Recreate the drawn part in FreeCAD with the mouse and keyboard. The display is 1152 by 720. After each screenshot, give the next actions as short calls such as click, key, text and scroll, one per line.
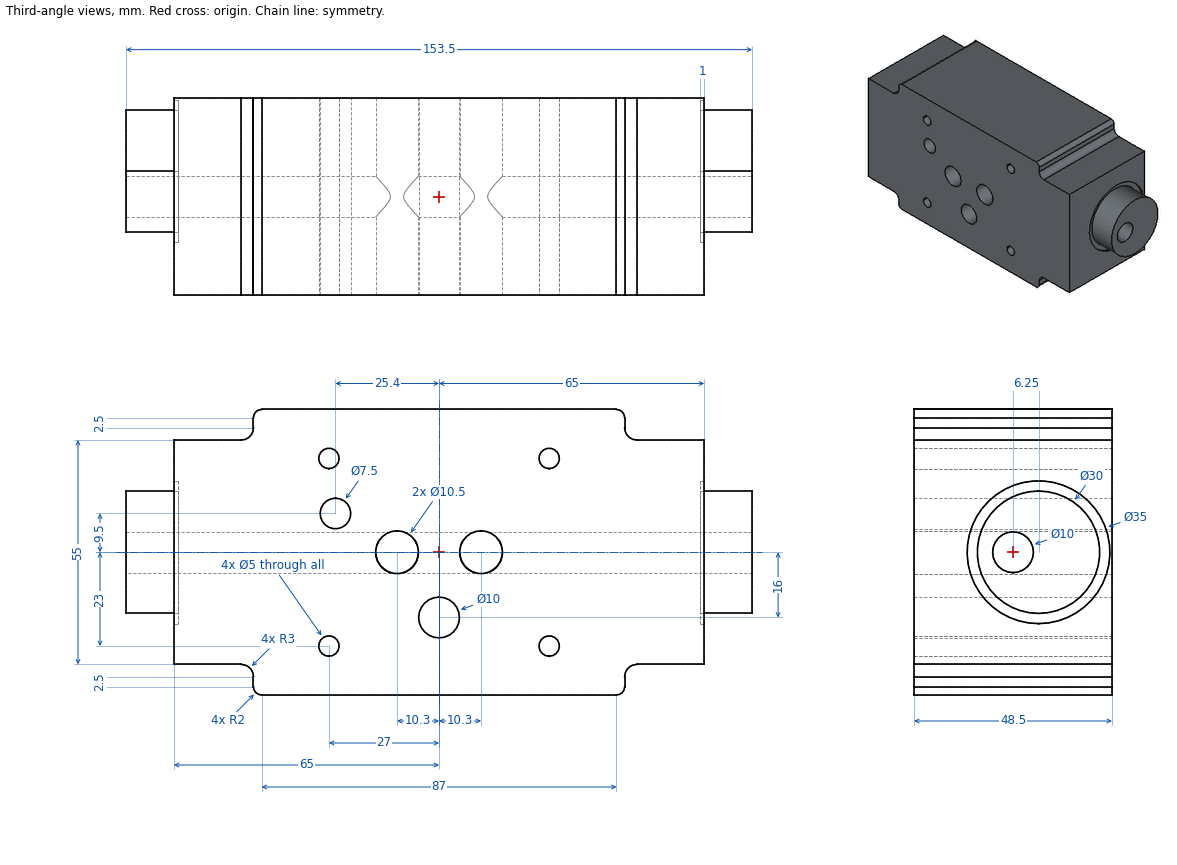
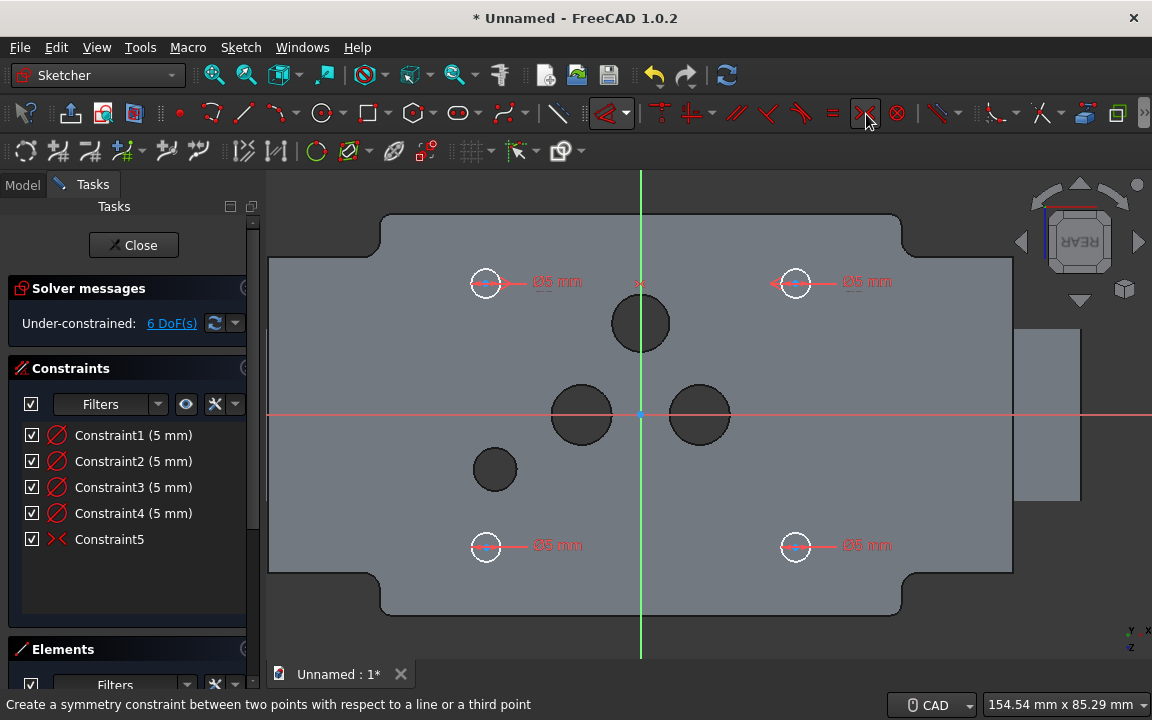
click(796, 284)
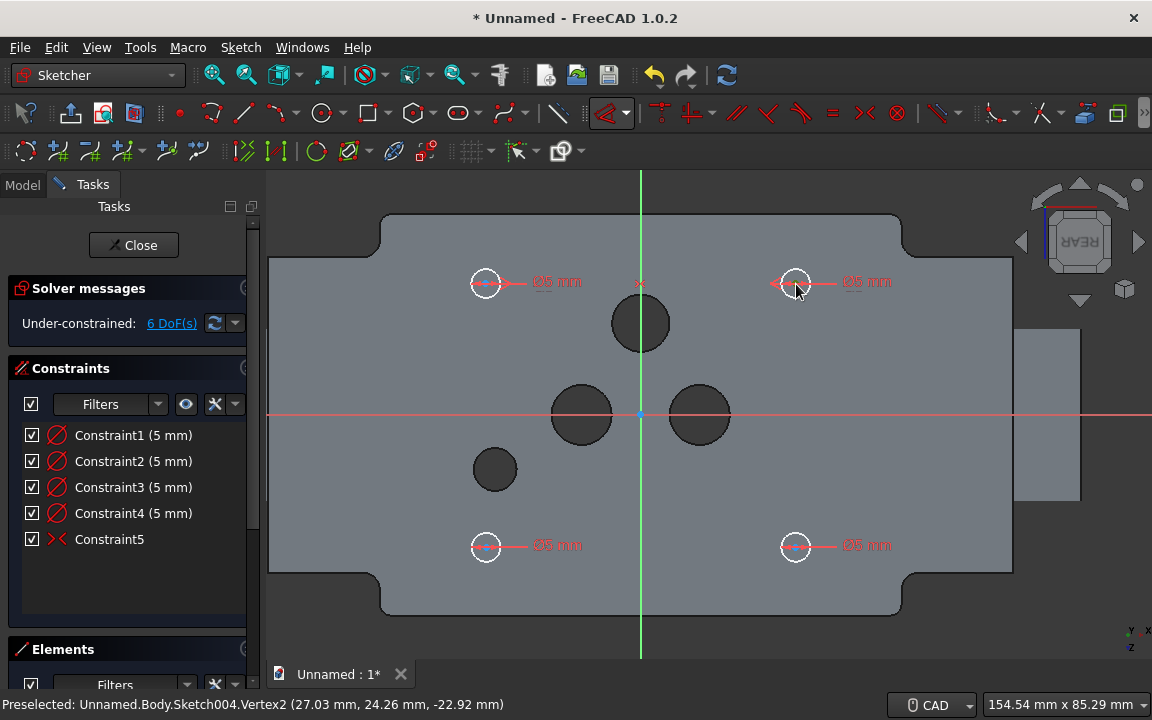
click(796, 547)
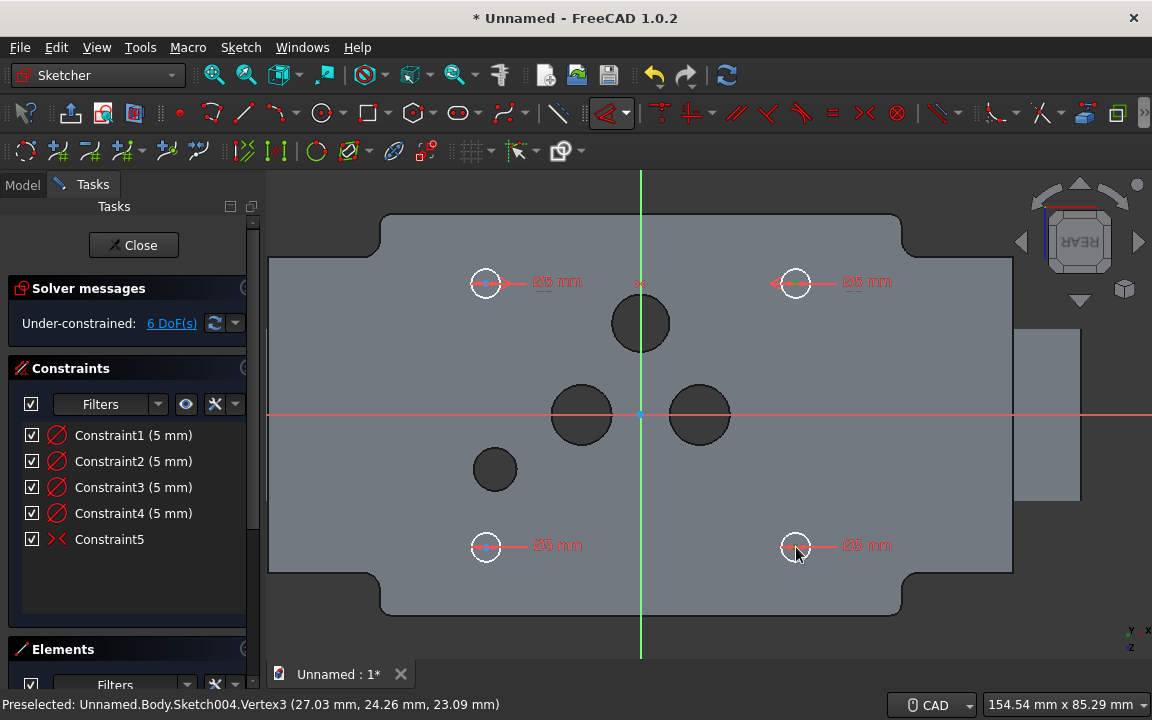
click(344, 415)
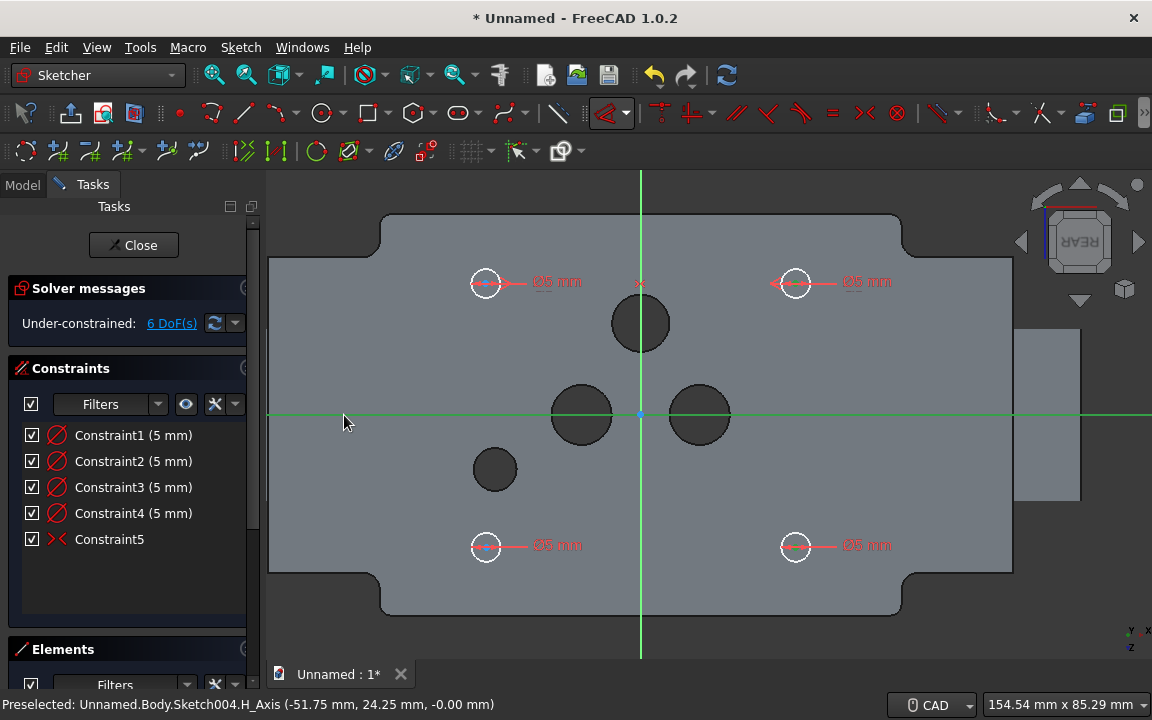
click(866, 114)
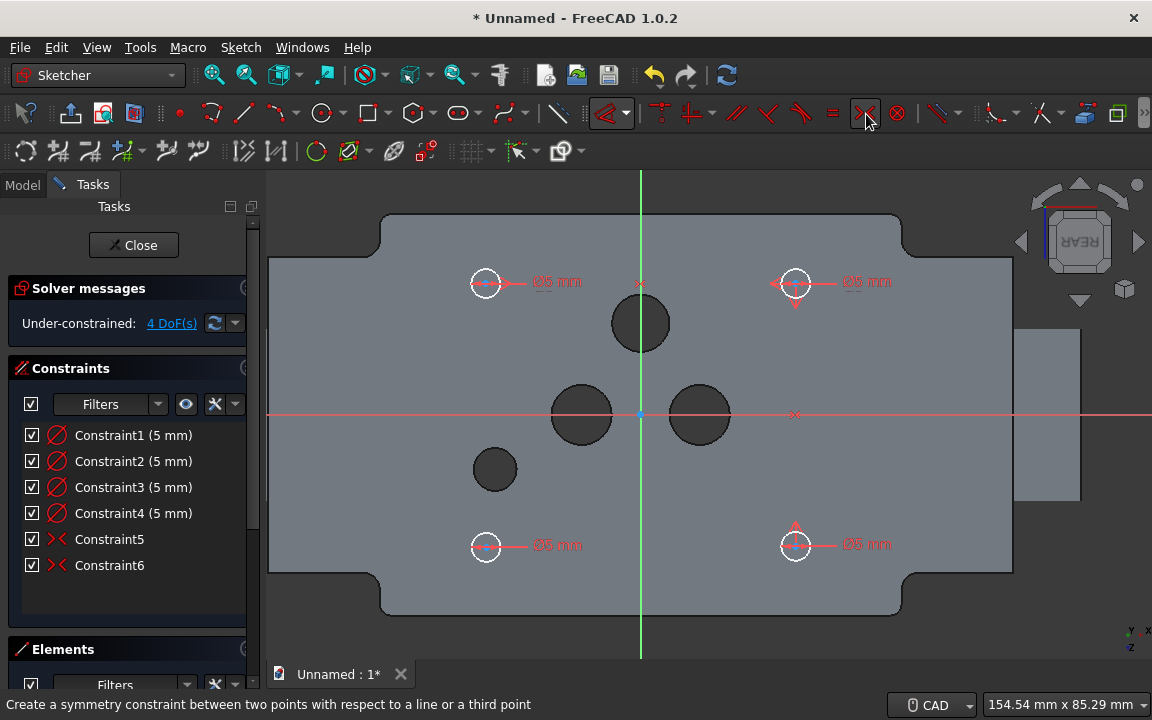
click(486, 284)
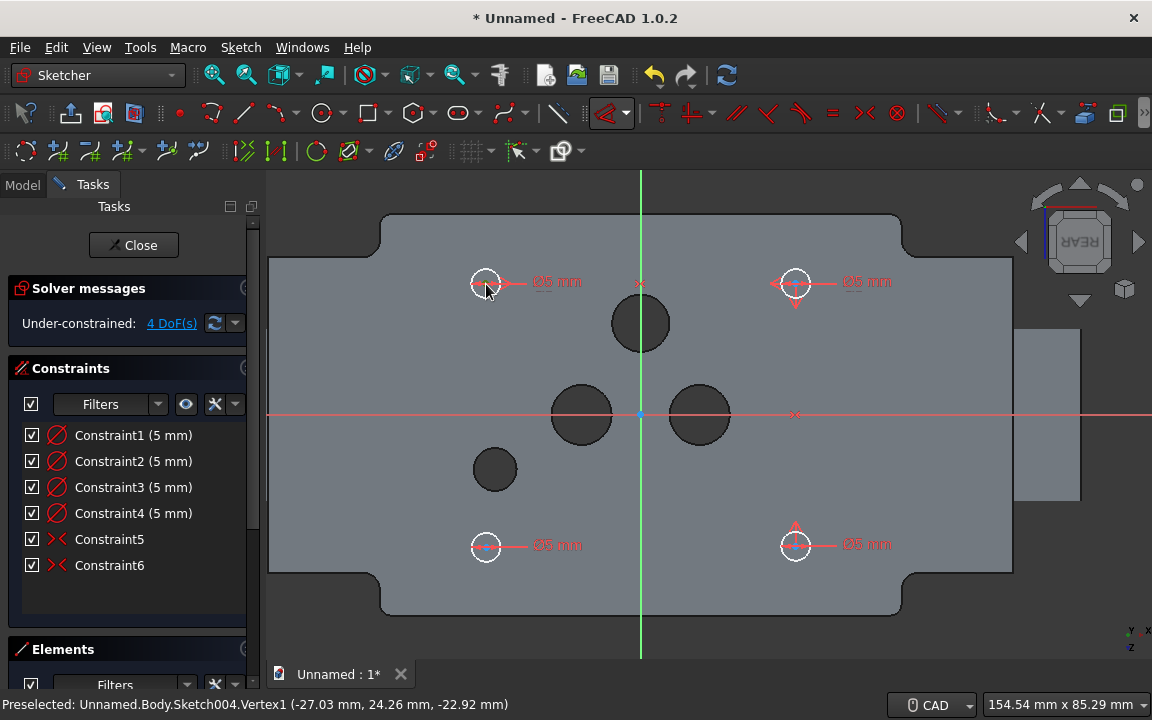
click(486, 547)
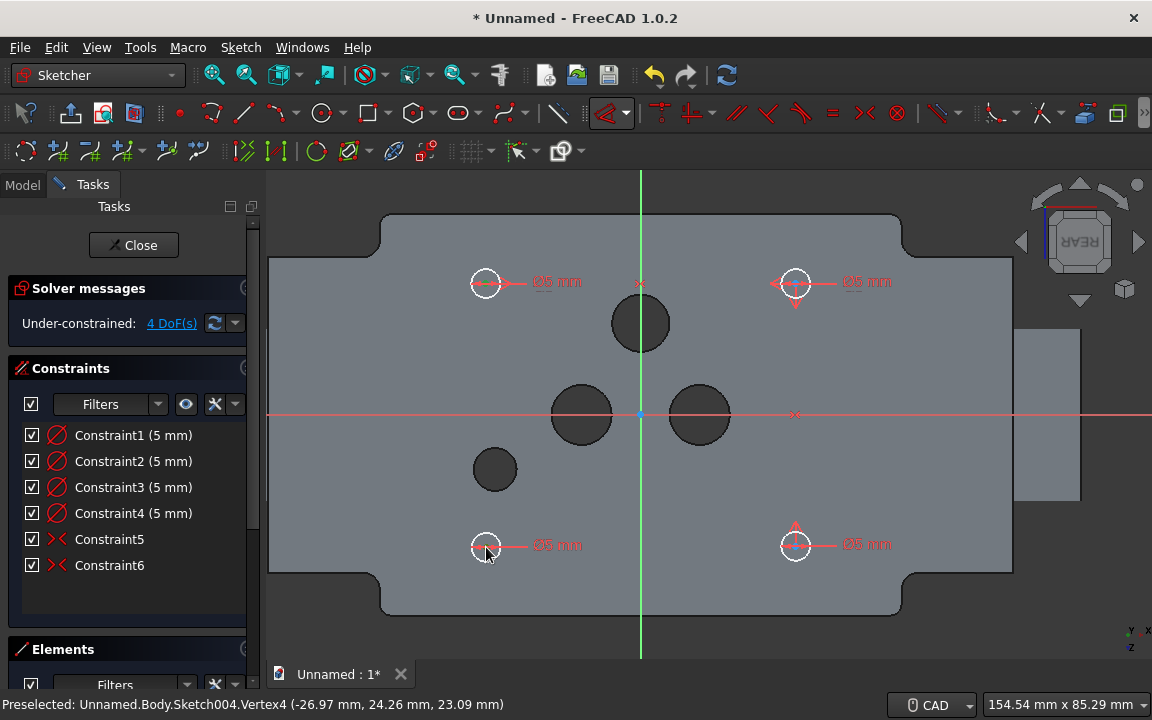
click(344, 415)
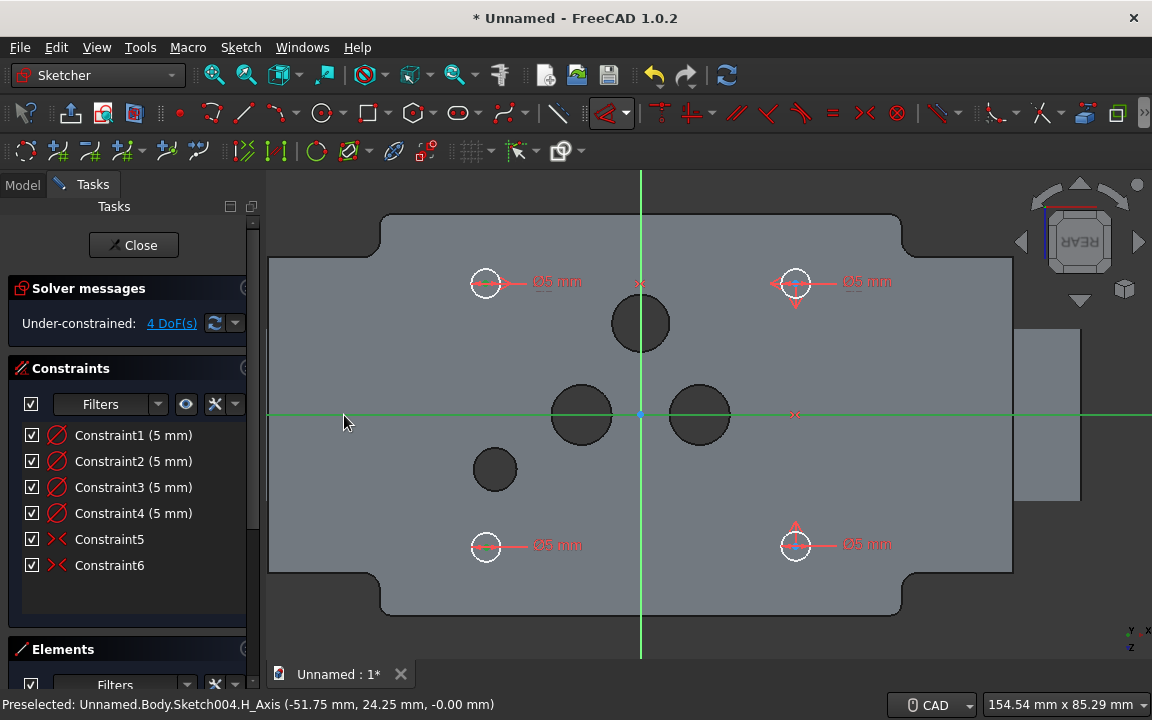
click(866, 114)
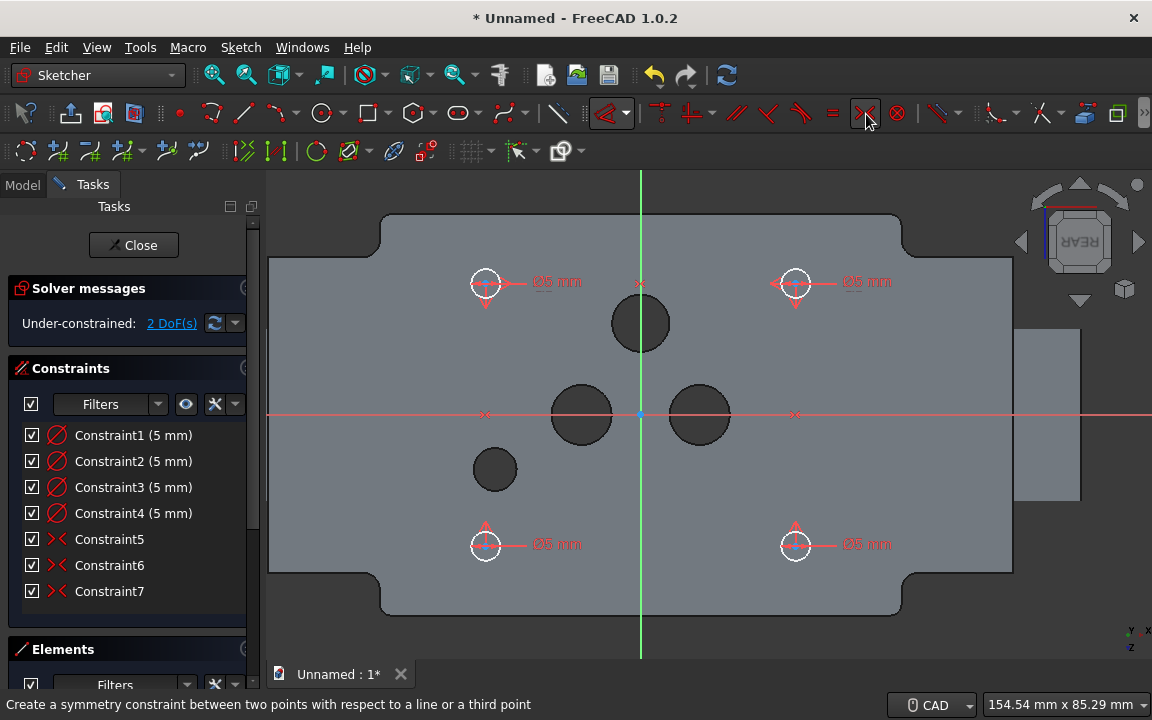
click(486, 284)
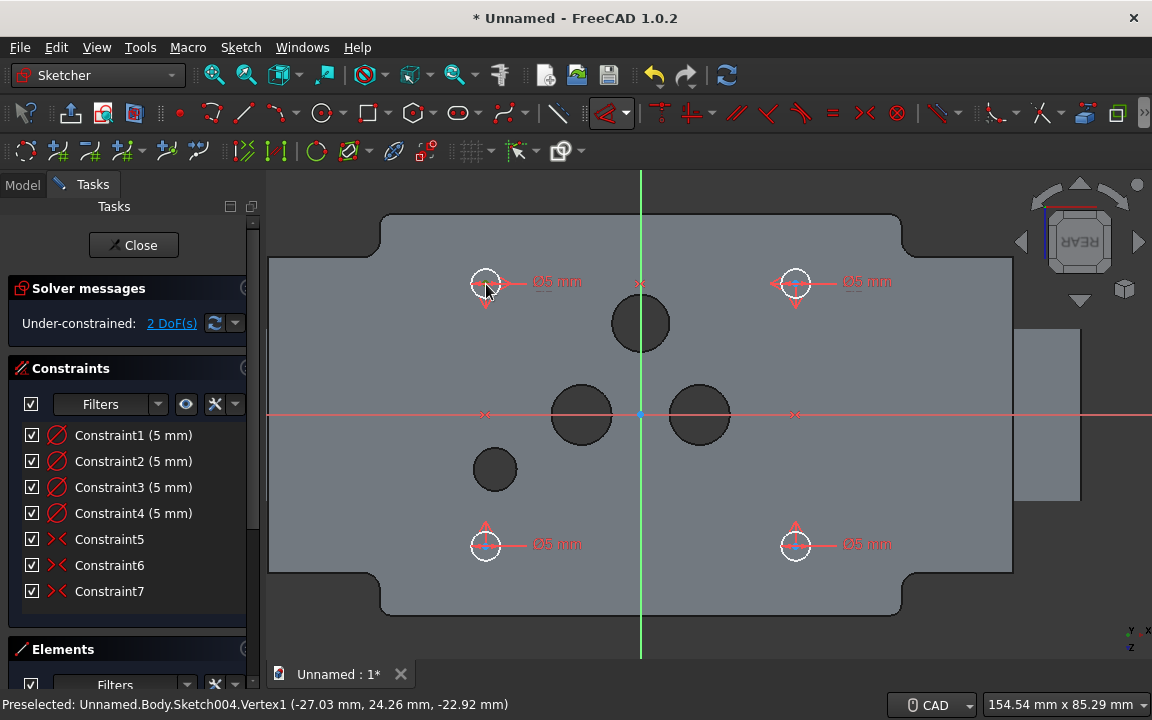
click(628, 114)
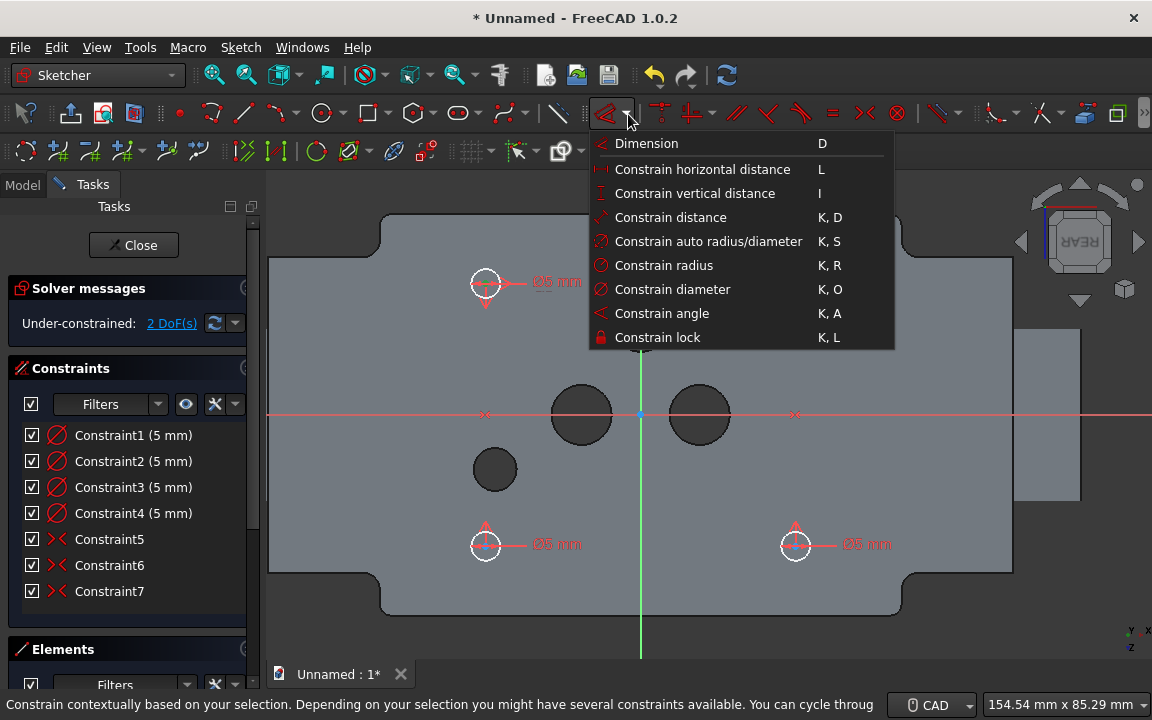
click(742, 169)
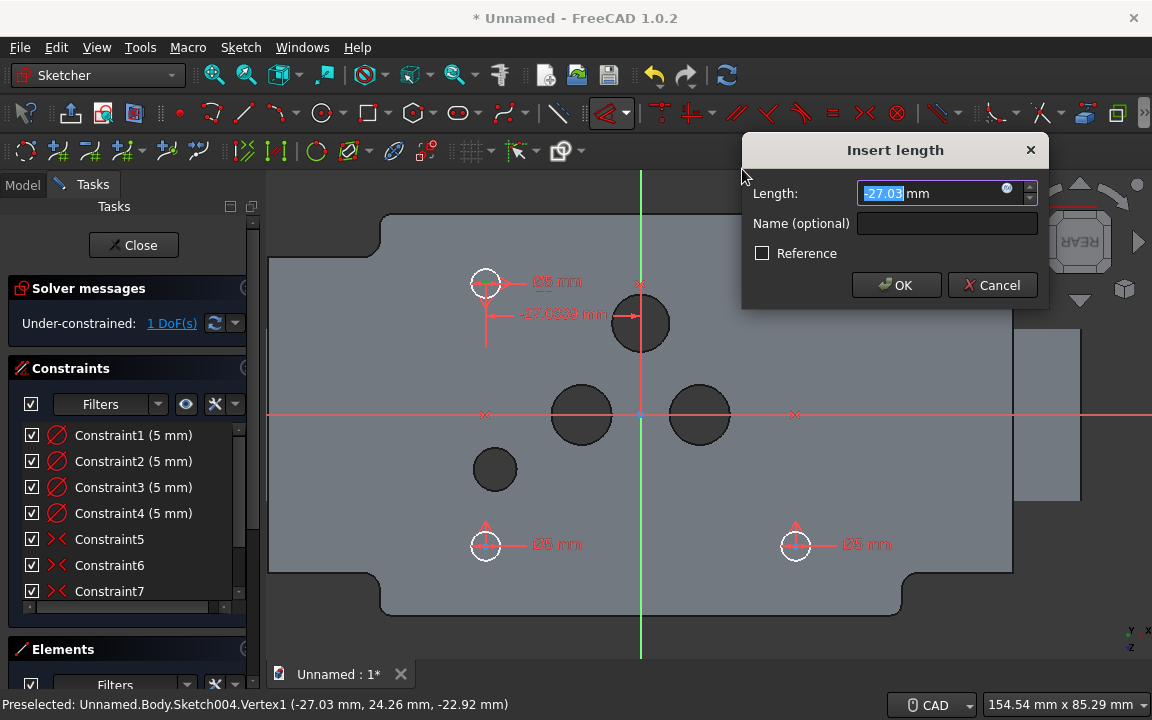
text(-27)
key(Return)